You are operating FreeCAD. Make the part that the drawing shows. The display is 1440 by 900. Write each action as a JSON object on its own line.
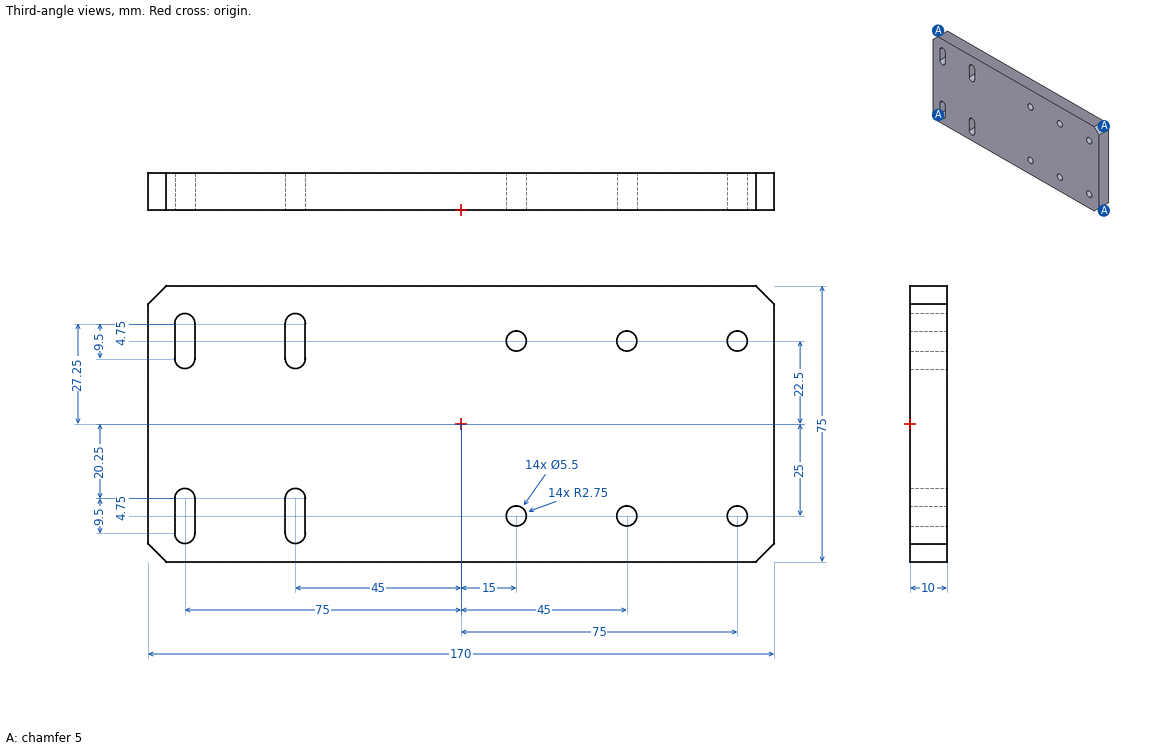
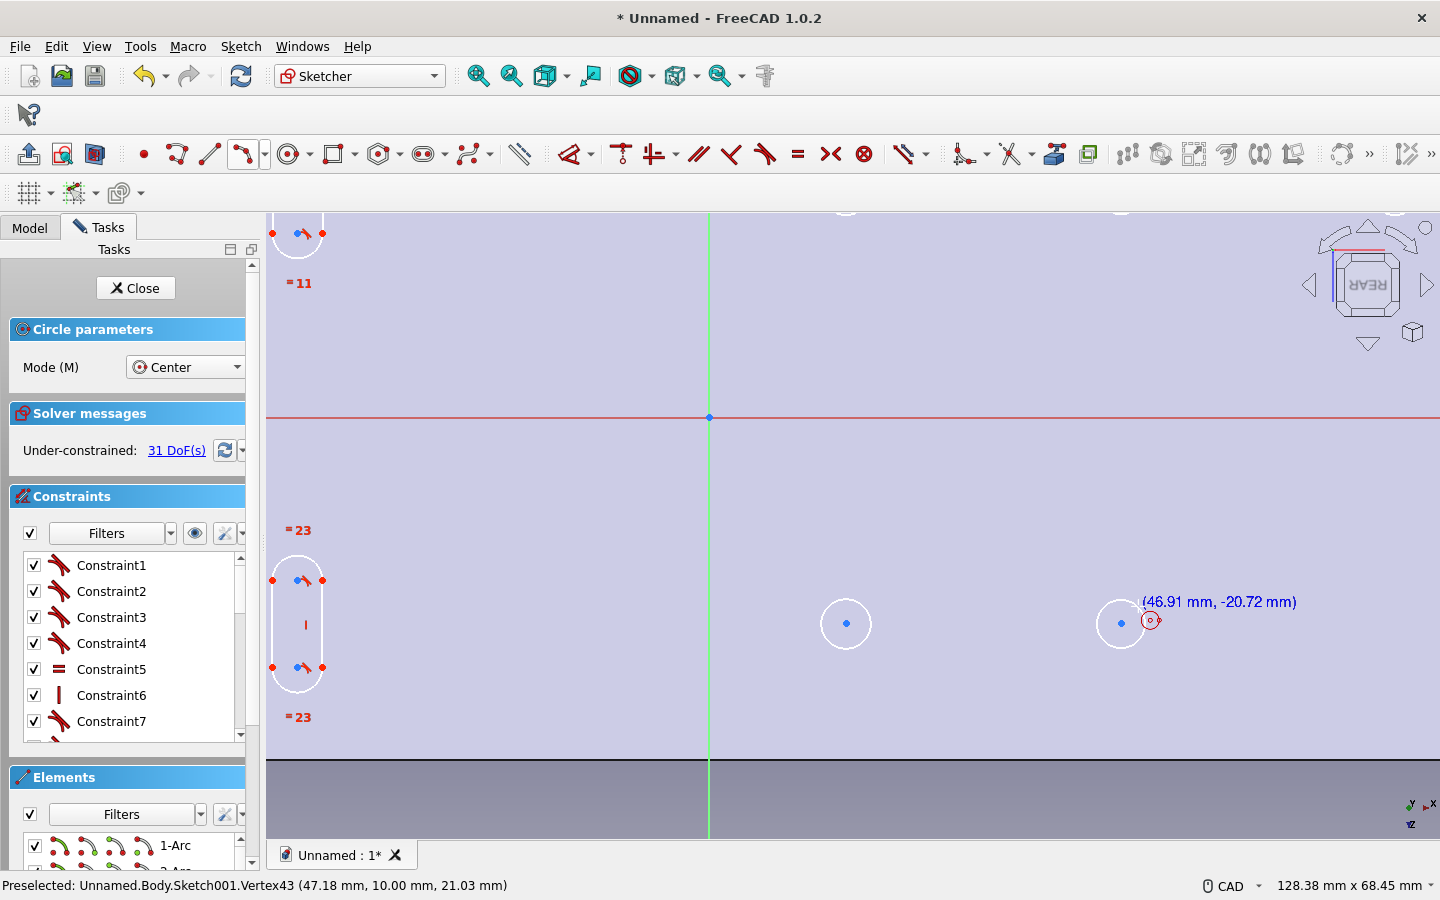
{"action": "scroll", "coordinate": [846, 624], "scroll_direction": "down", "scroll_amount": 4}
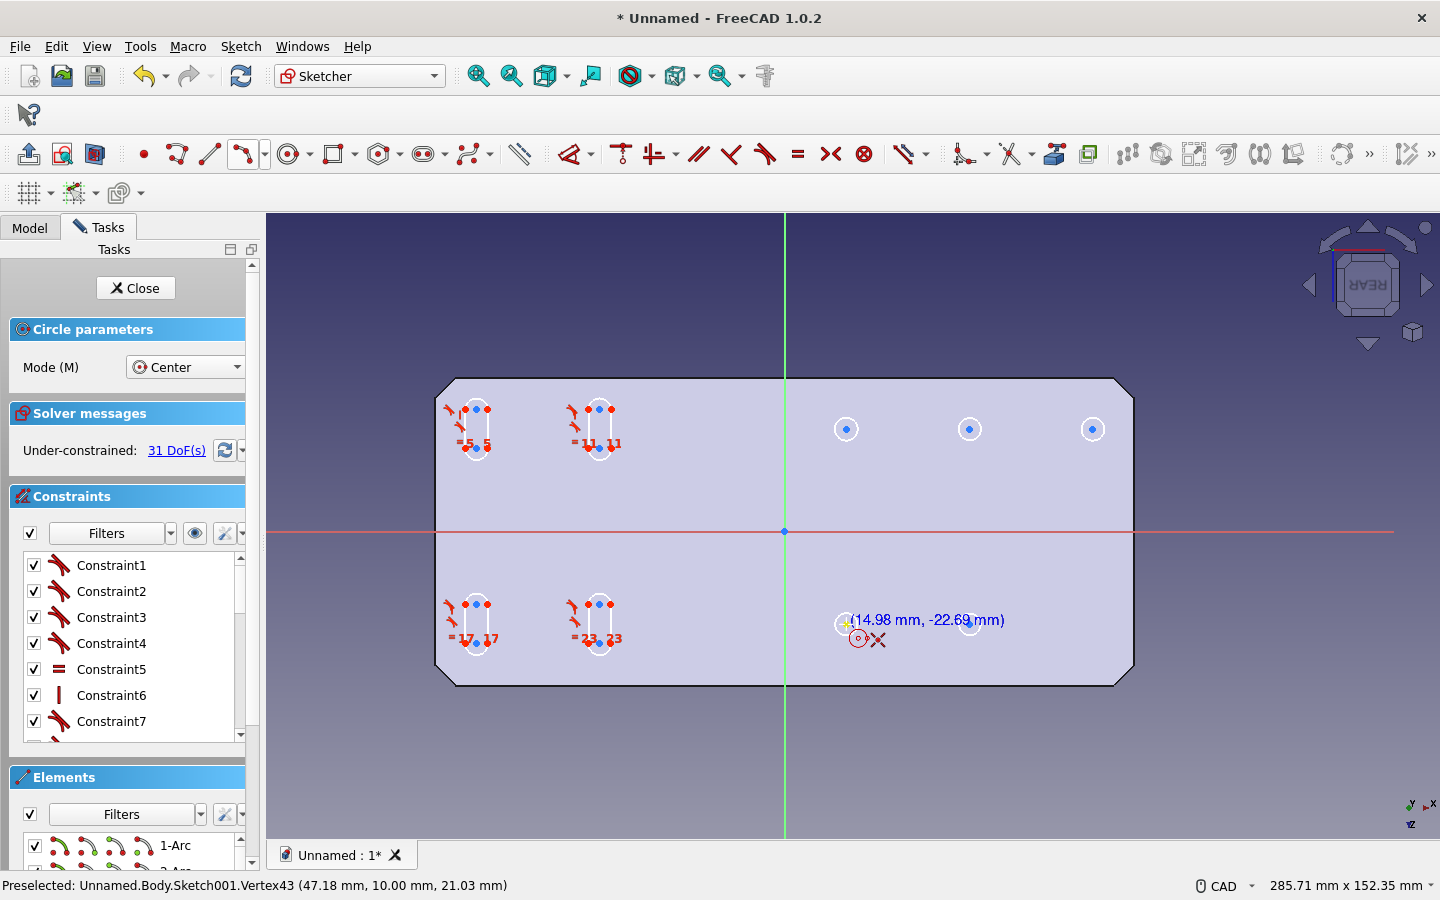
{"action": "scroll", "coordinate": [1093, 624], "scroll_direction": "up", "scroll_amount": 4}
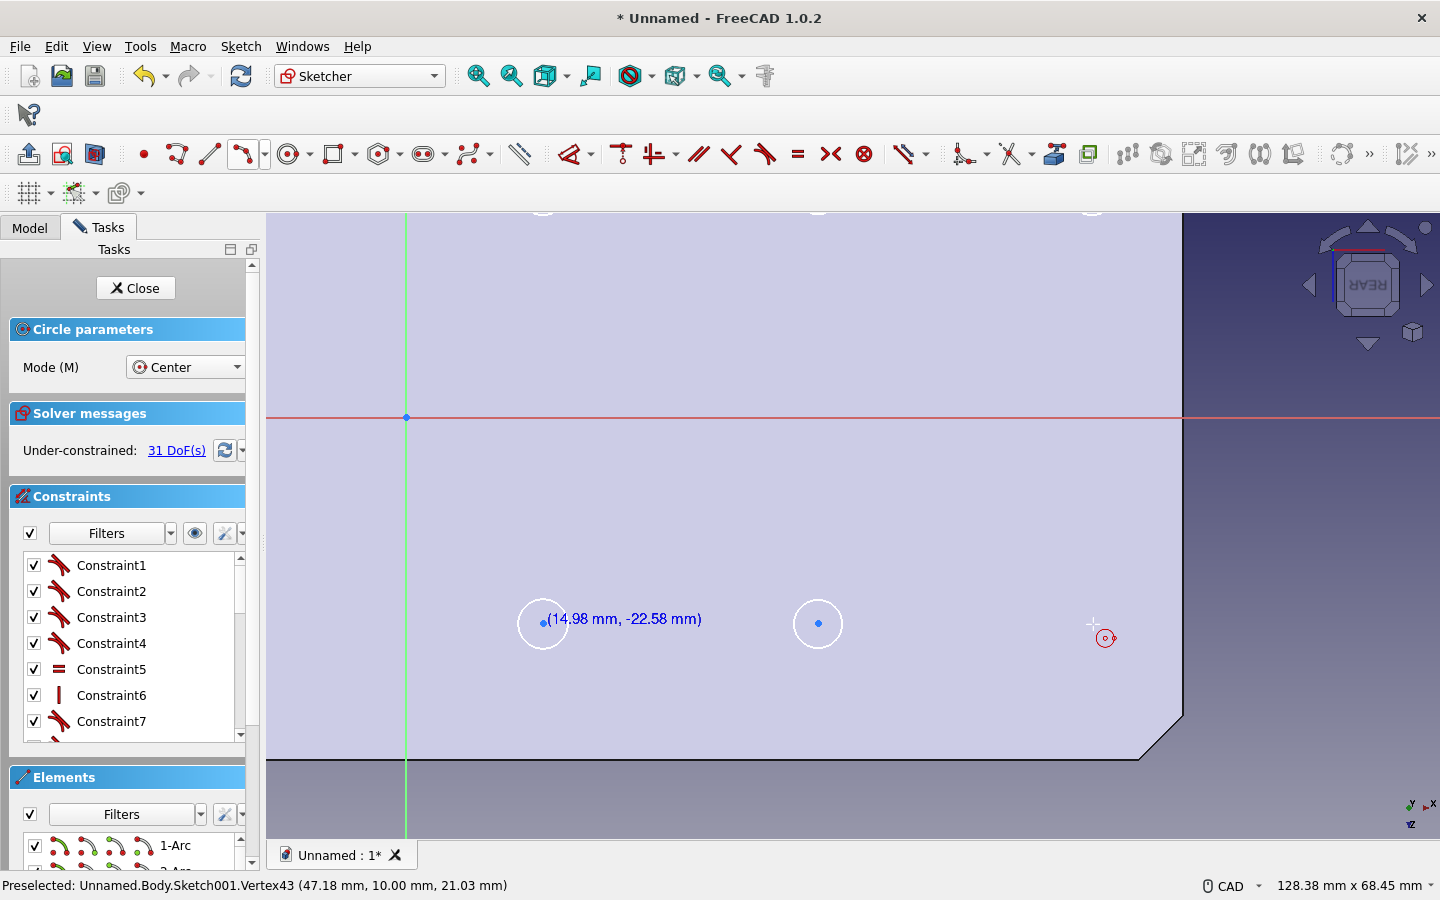
{"action": "left_click", "coordinate": [1092, 623]}
{"action": "left_click", "coordinate": [1110, 606]}
{"action": "key", "text": "Escape"}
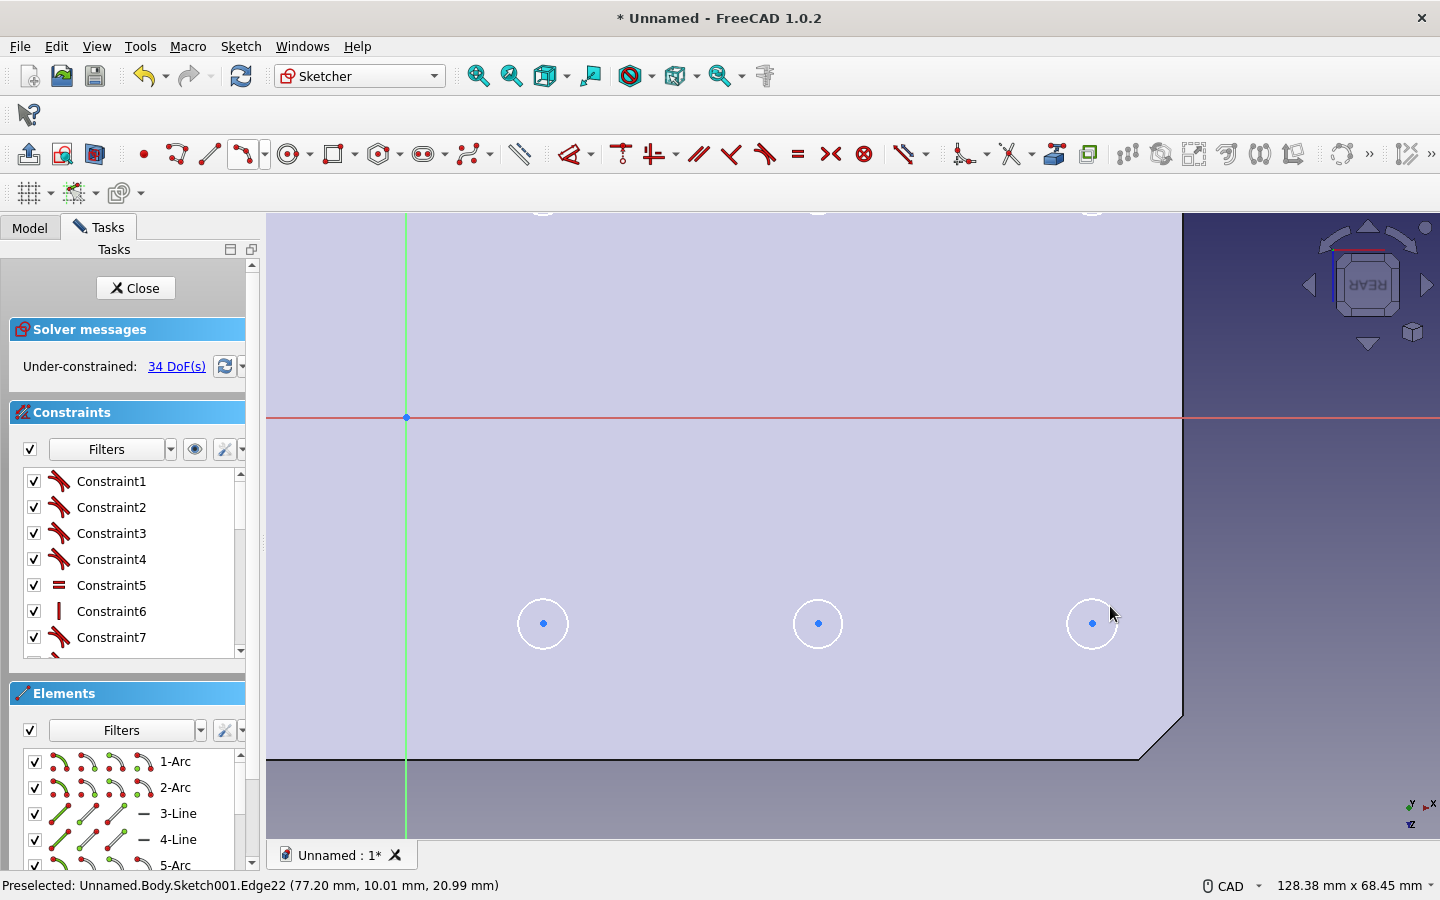
{"action": "scroll", "coordinate": [1093, 624], "scroll_direction": "down", "scroll_amount": 4}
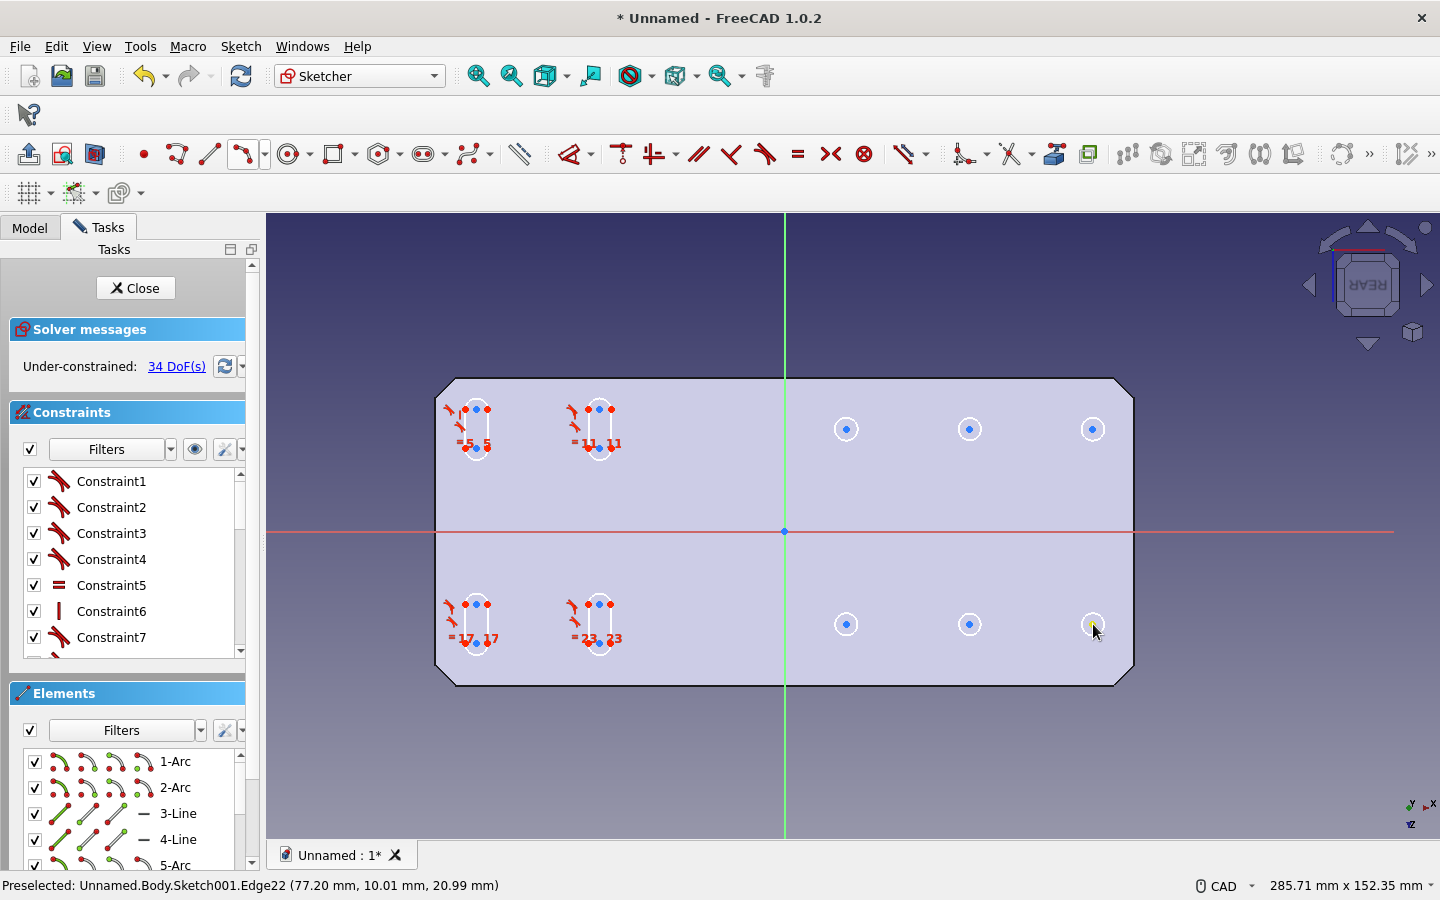
{"action": "scroll", "coordinate": [470, 458], "scroll_direction": "up", "scroll_amount": 2}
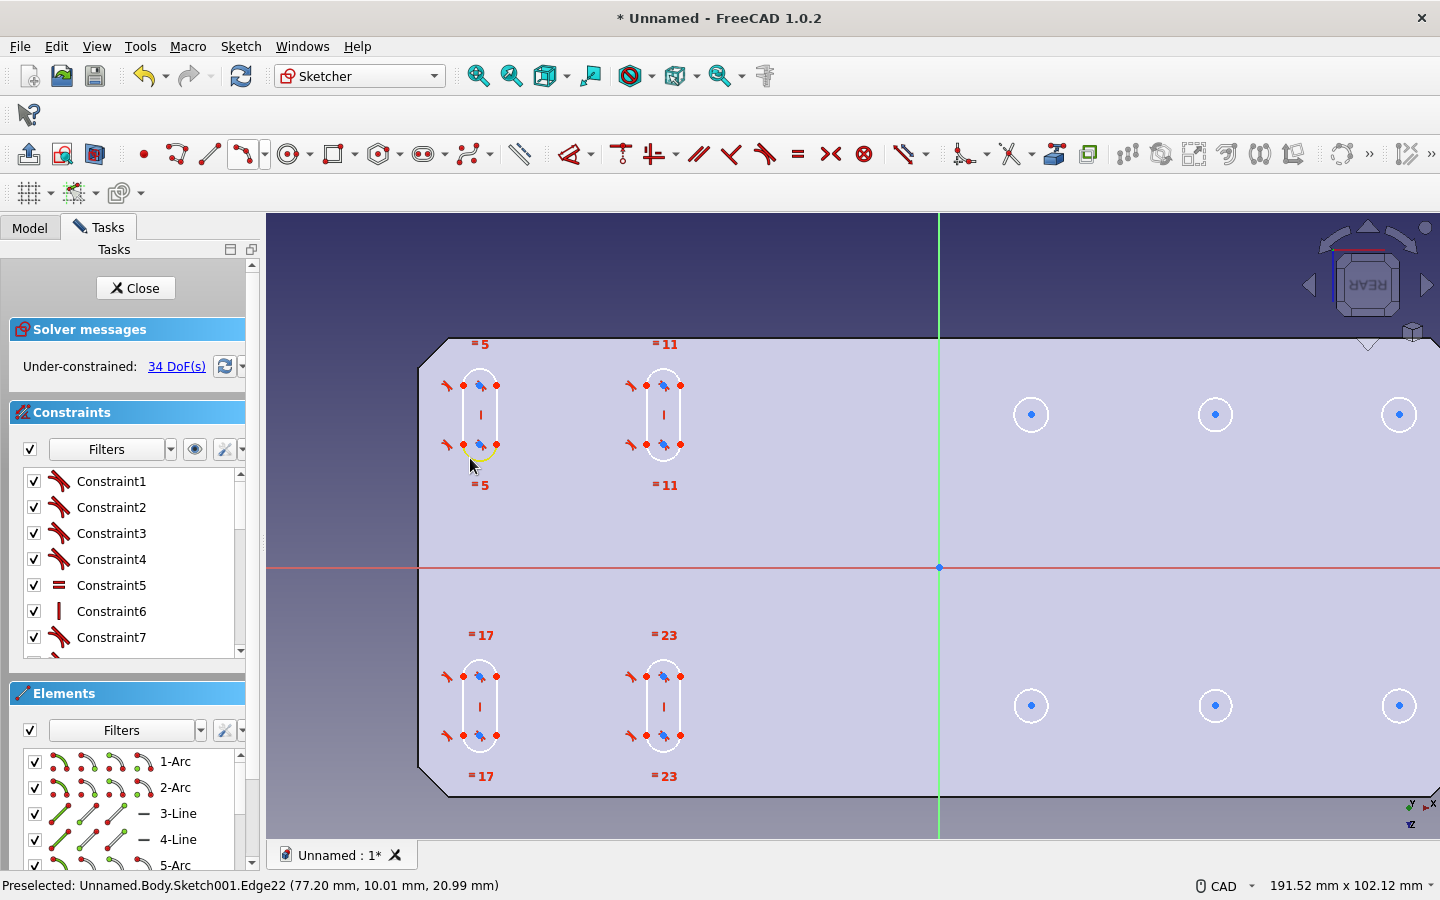
{"action": "left_click", "coordinate": [470, 458]}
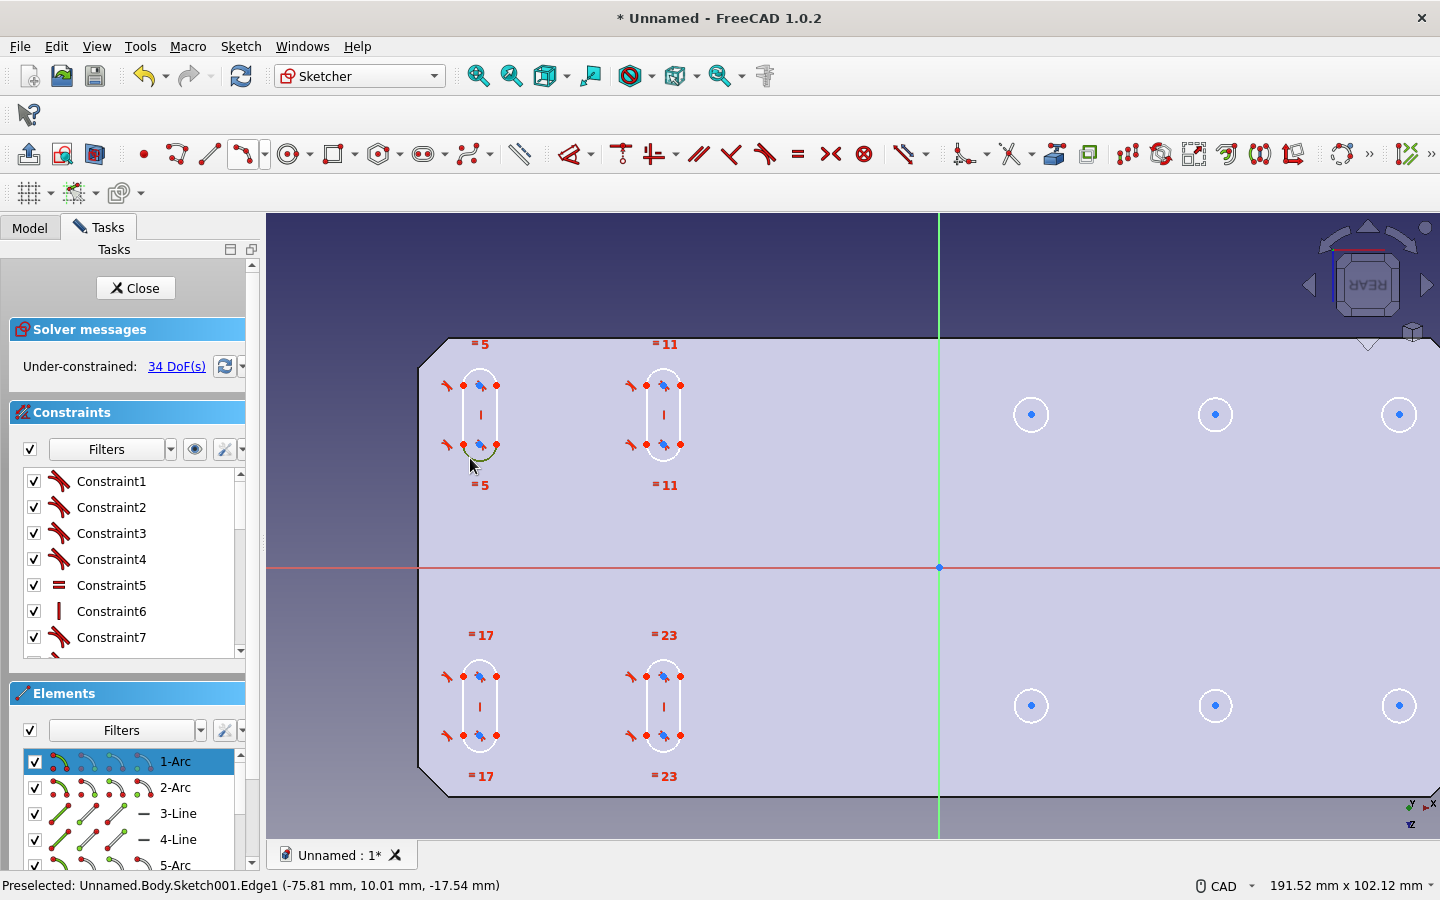
{"action": "left_click", "coordinate": [654, 458]}